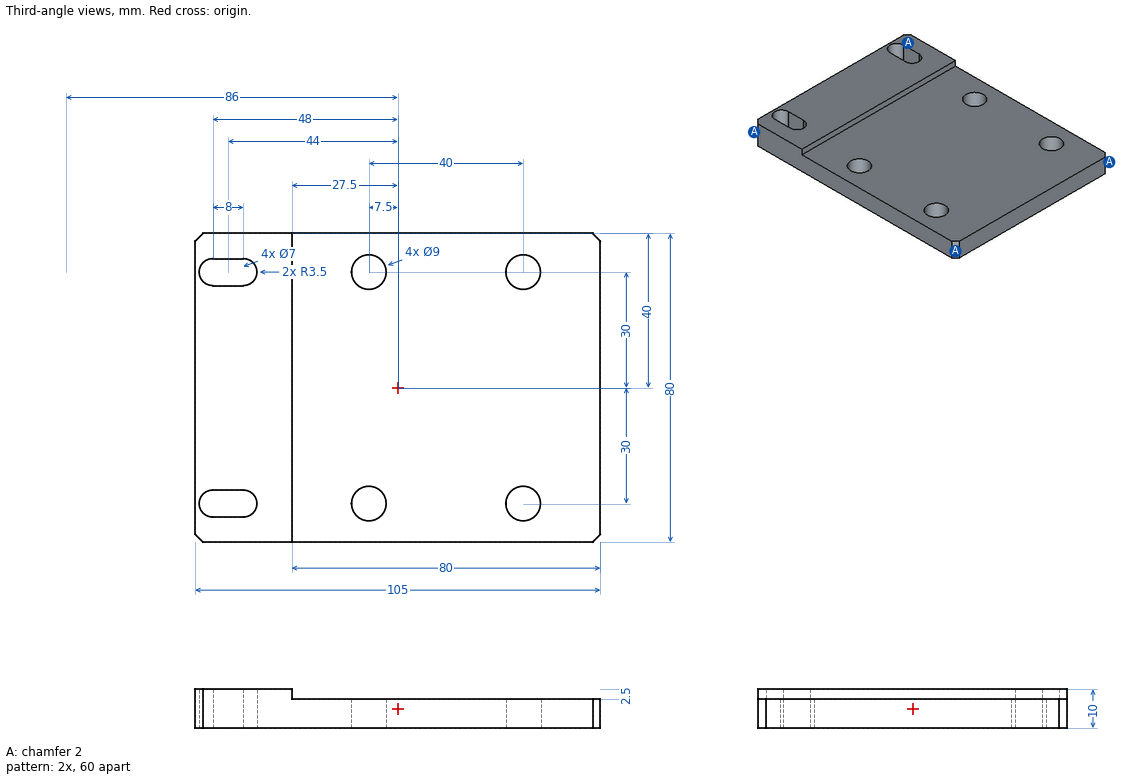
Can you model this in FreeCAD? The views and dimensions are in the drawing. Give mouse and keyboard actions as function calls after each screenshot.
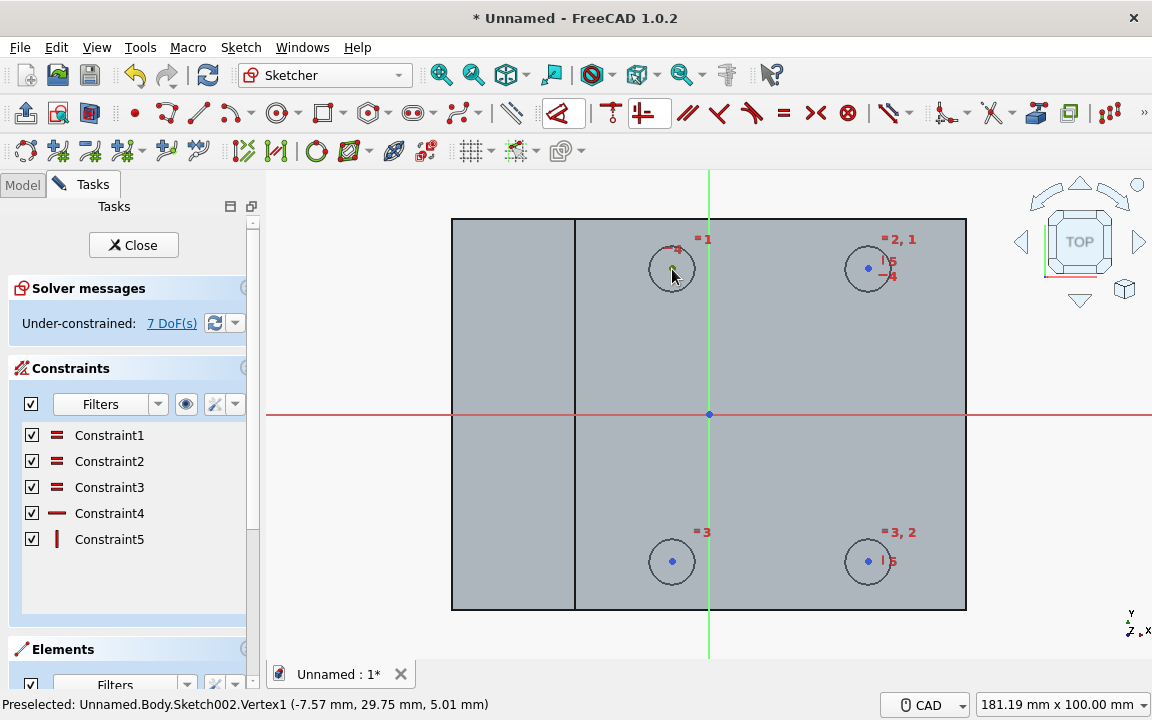
click(672, 562)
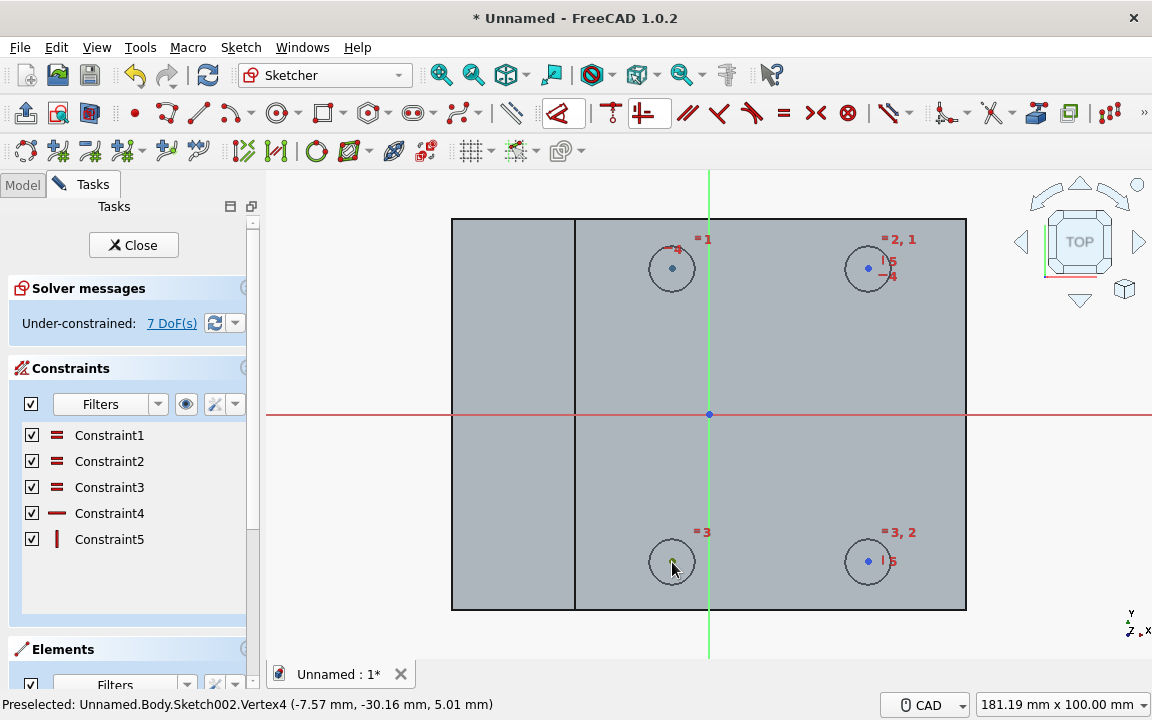
key(v)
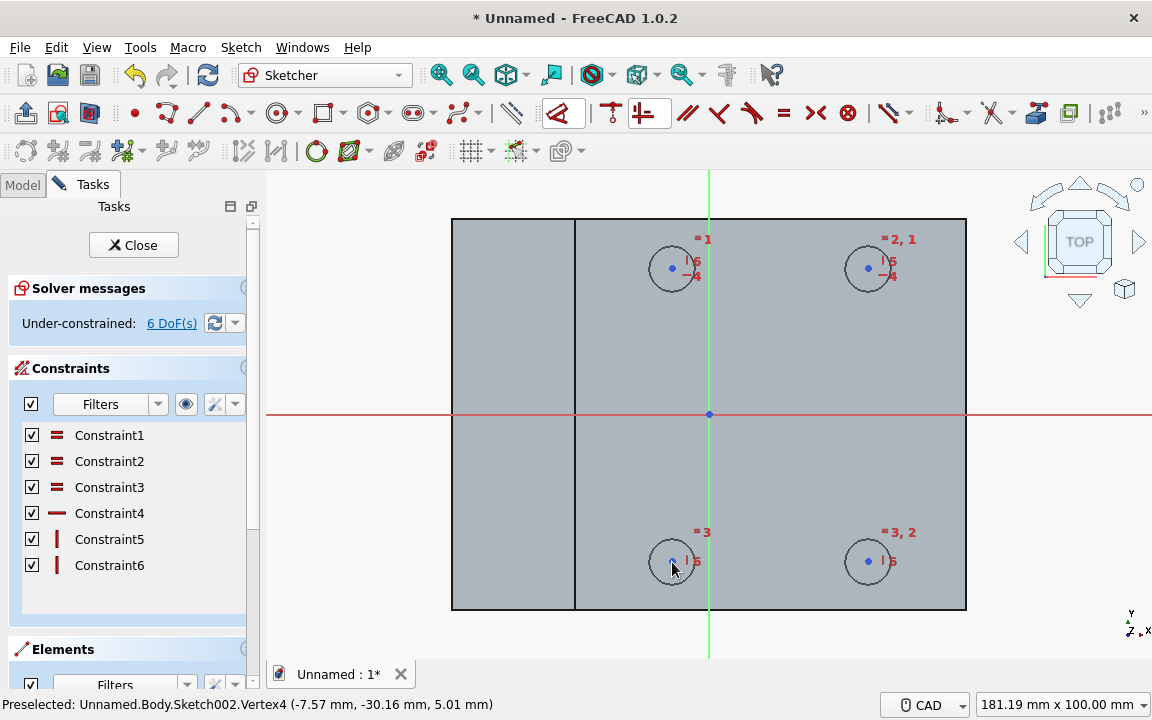
click(868, 562)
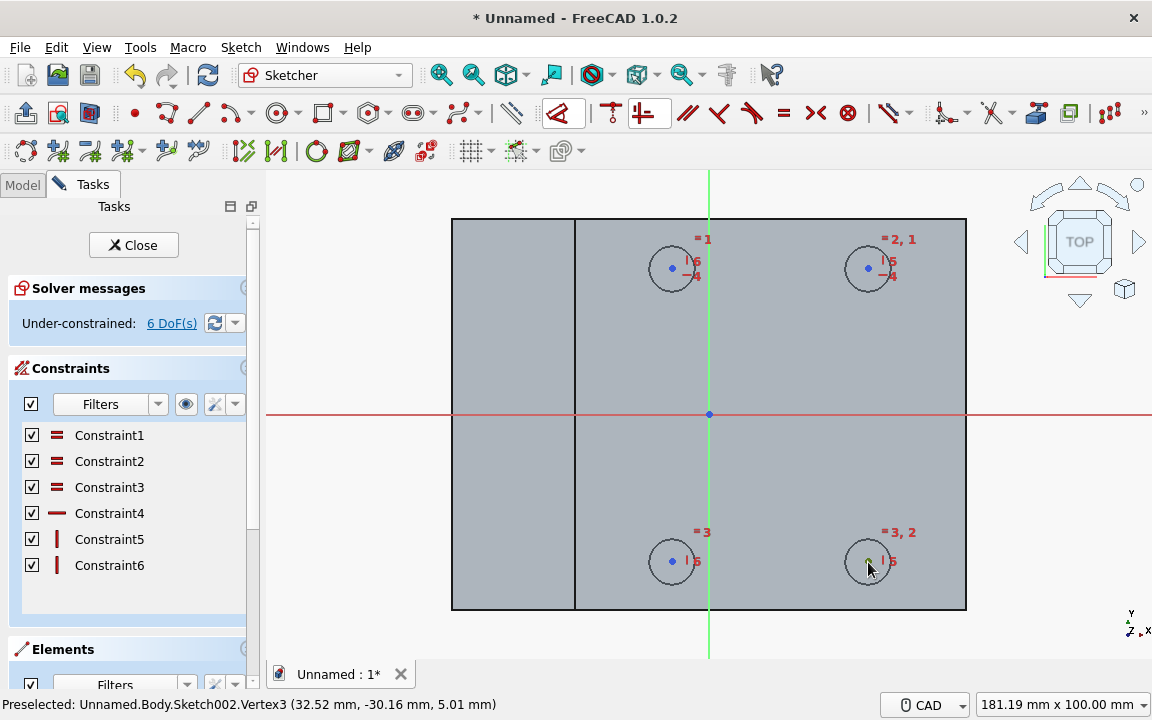
click(672, 562)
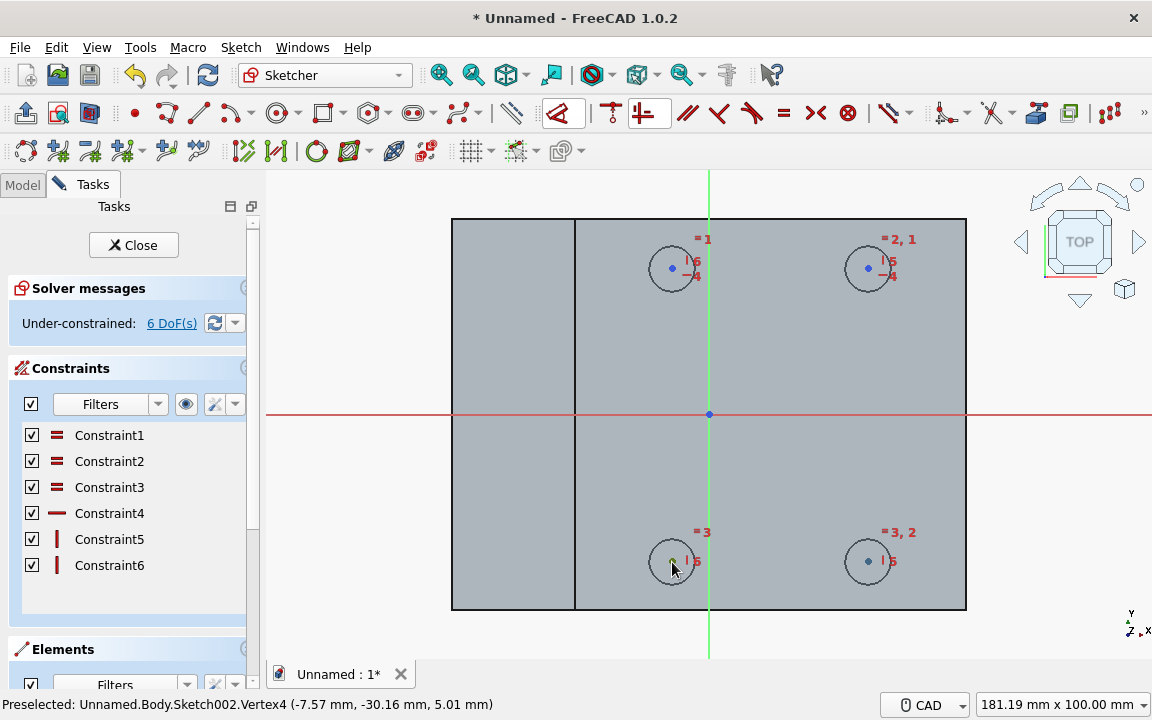
key(h)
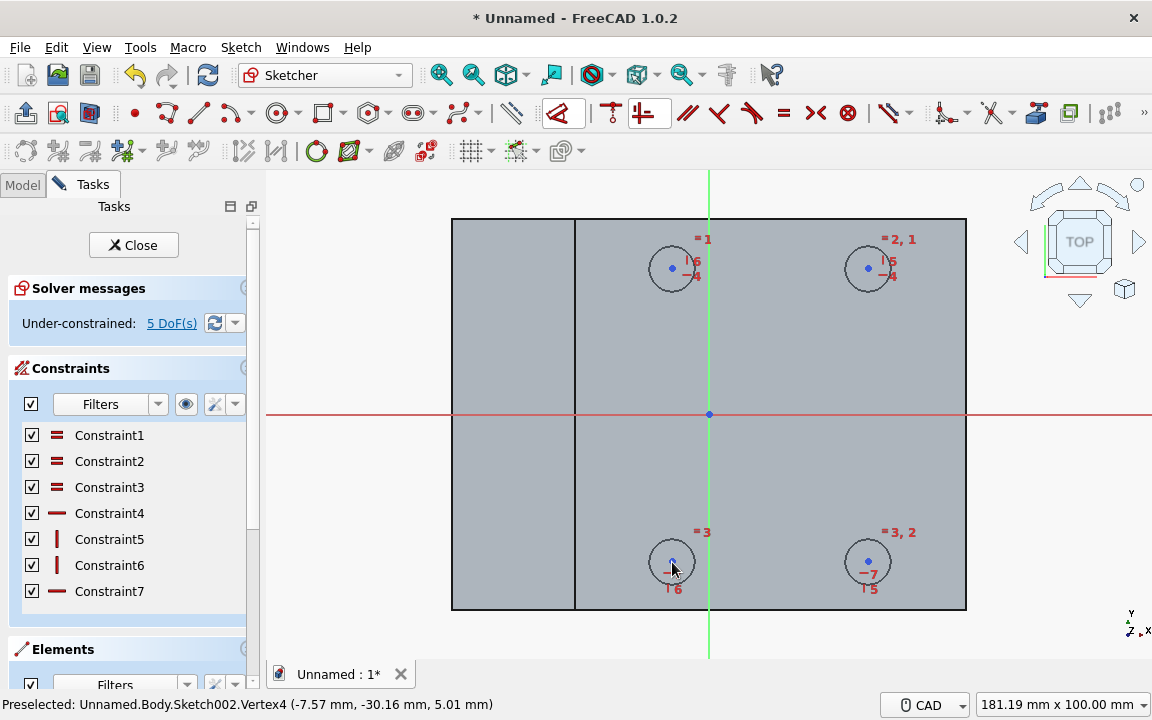
click(656, 253)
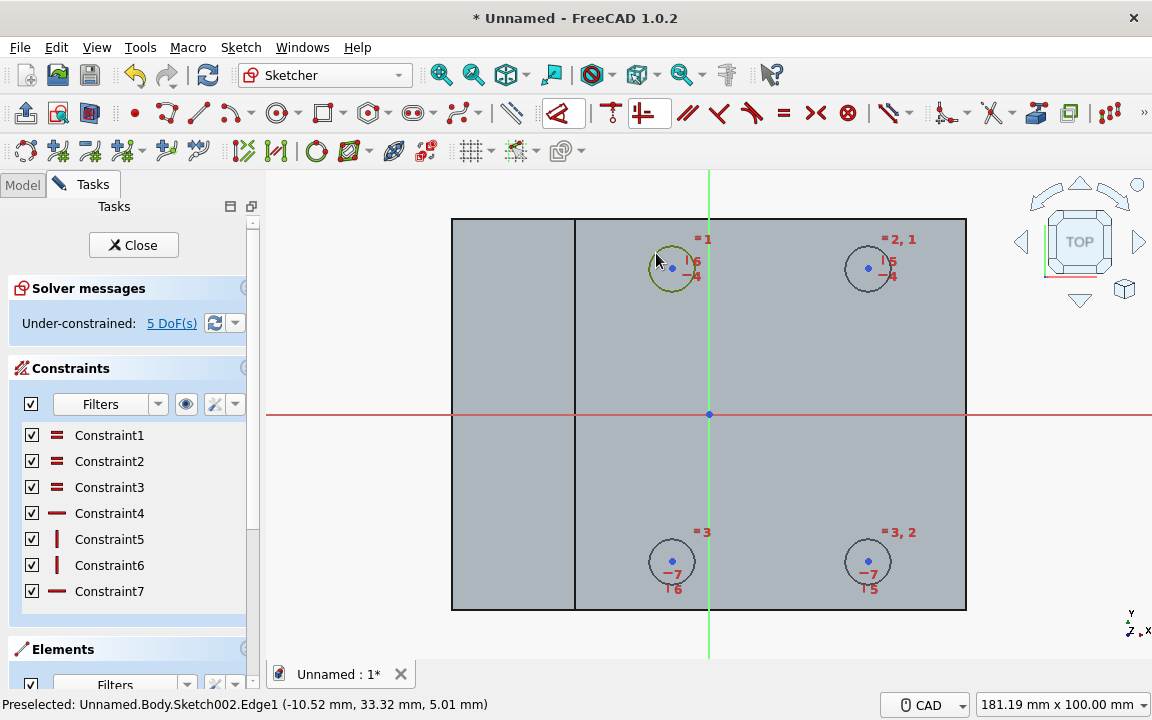
key(k)
key(o)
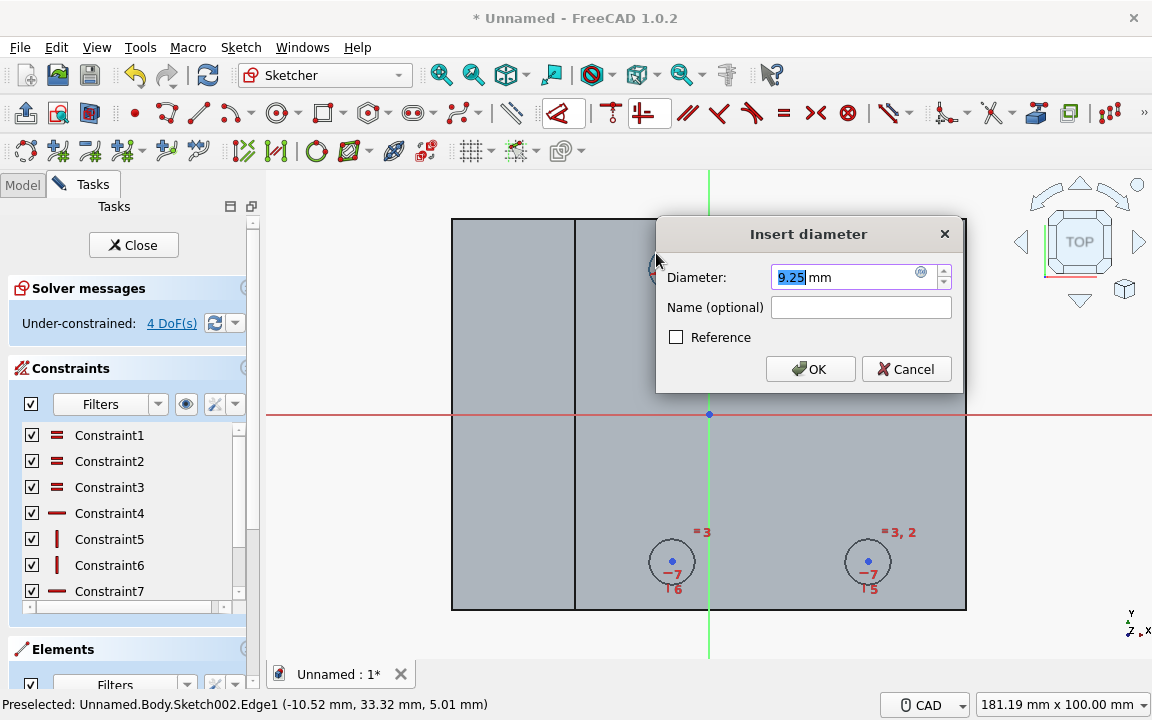
text(9)
key(Return)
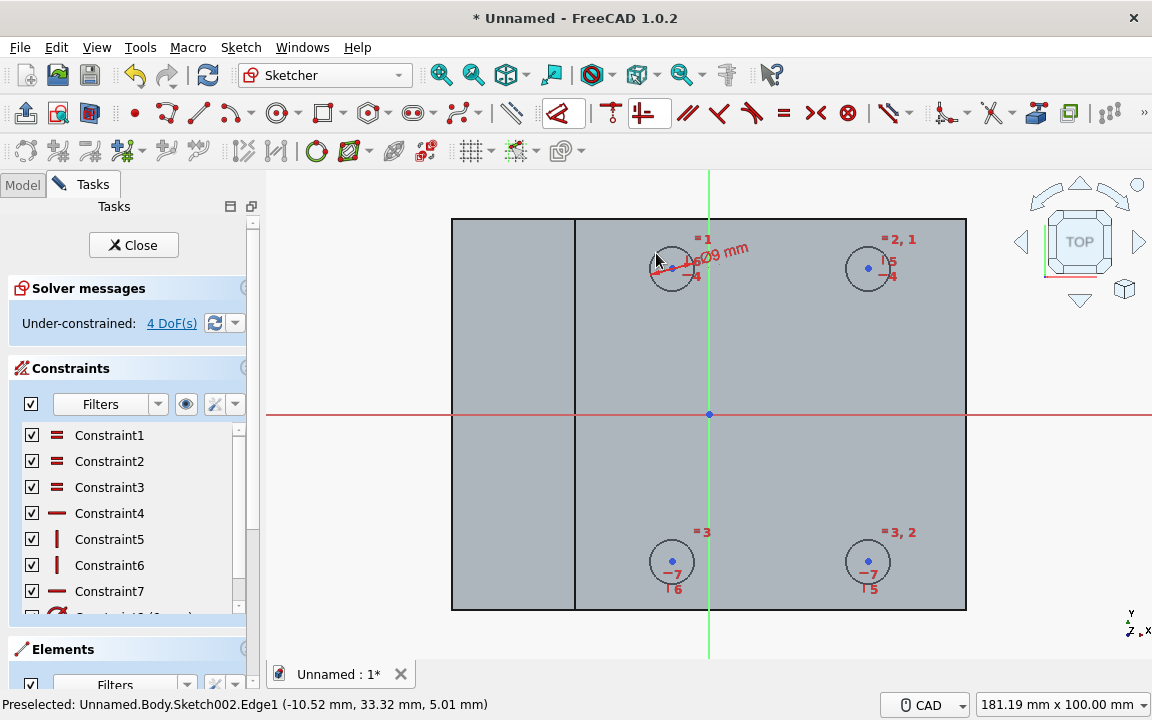
click(672, 269)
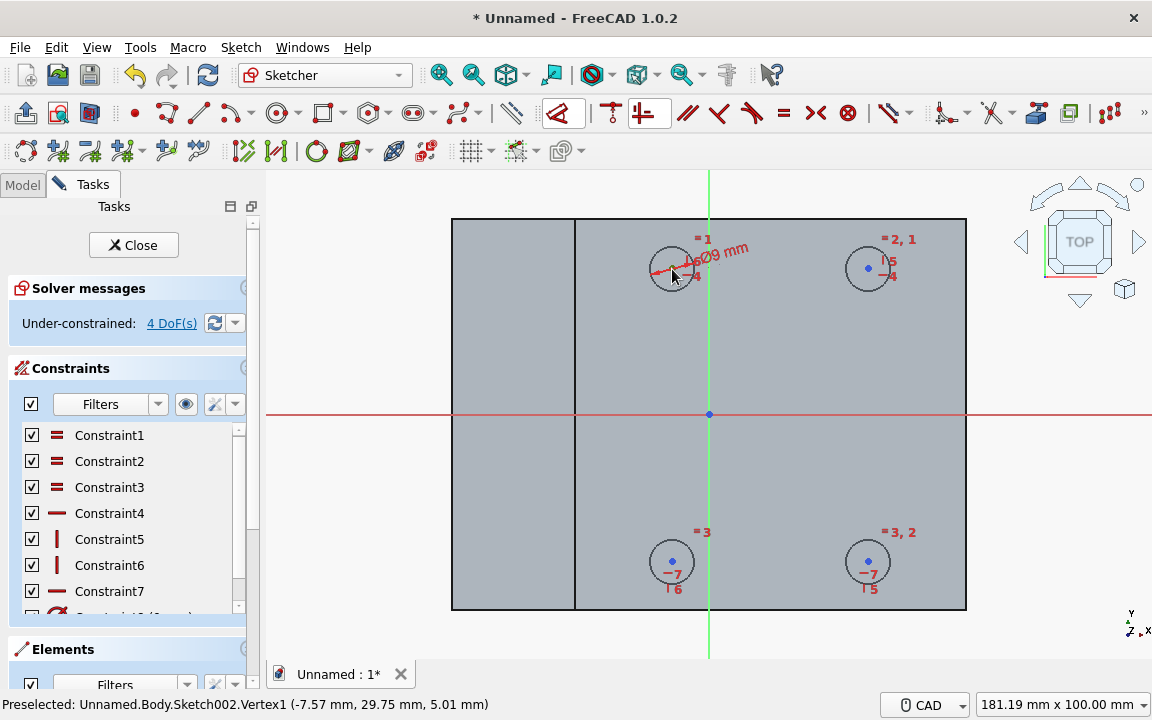
key(i)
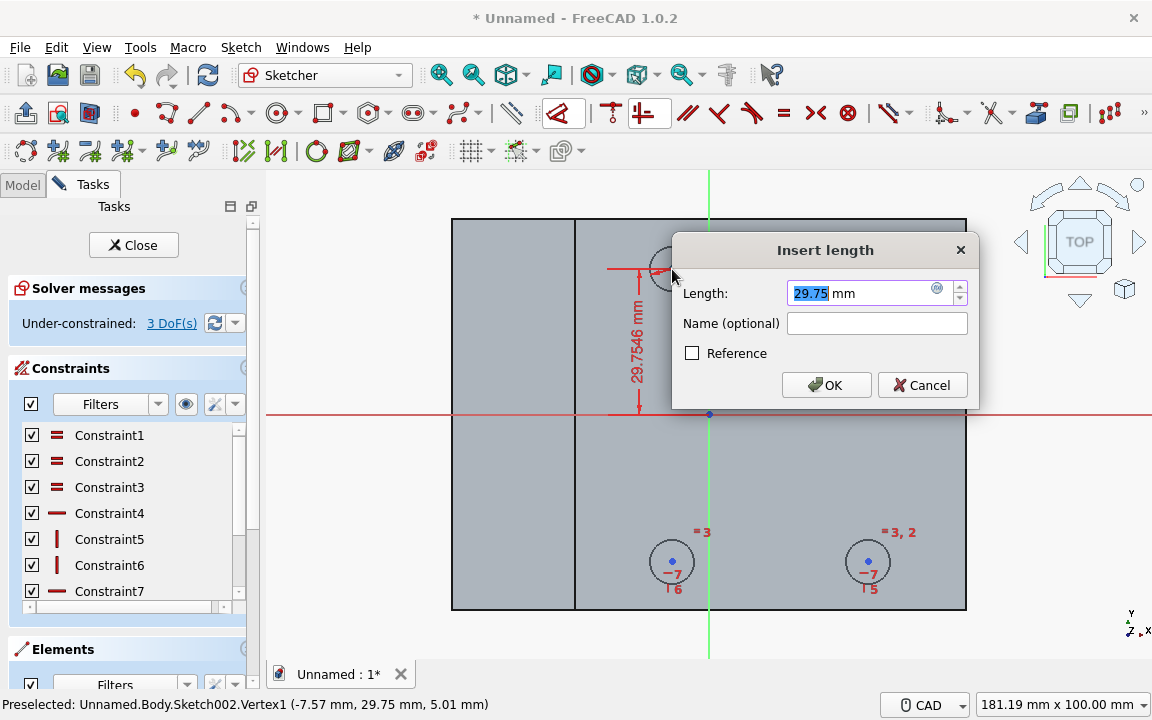
text(30)
key(Return)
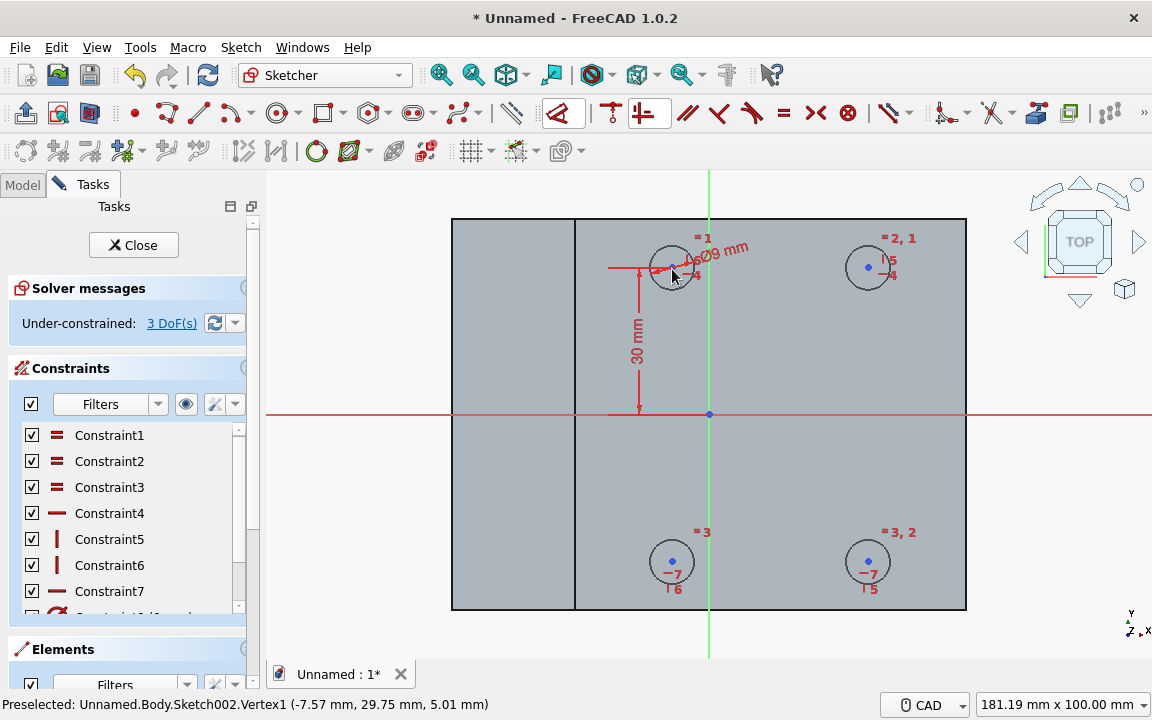
click(868, 562)